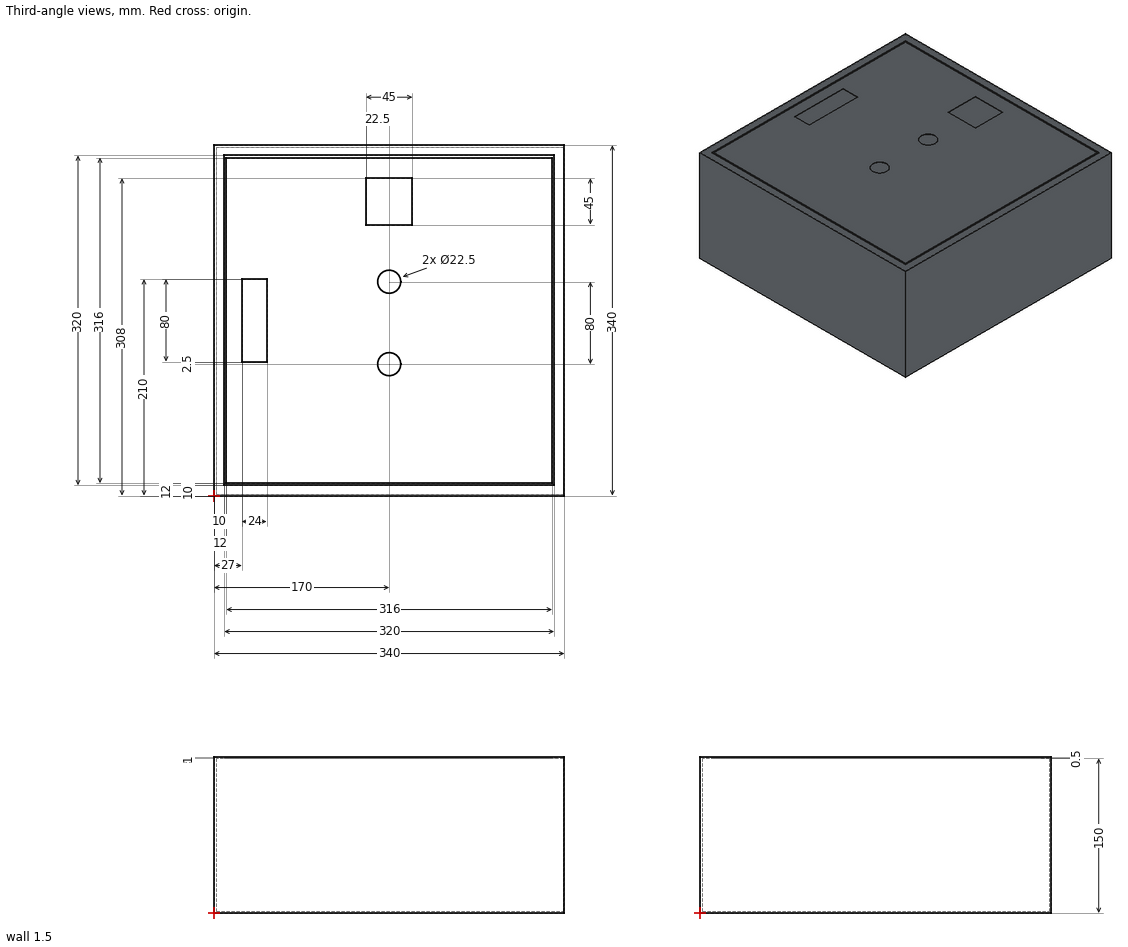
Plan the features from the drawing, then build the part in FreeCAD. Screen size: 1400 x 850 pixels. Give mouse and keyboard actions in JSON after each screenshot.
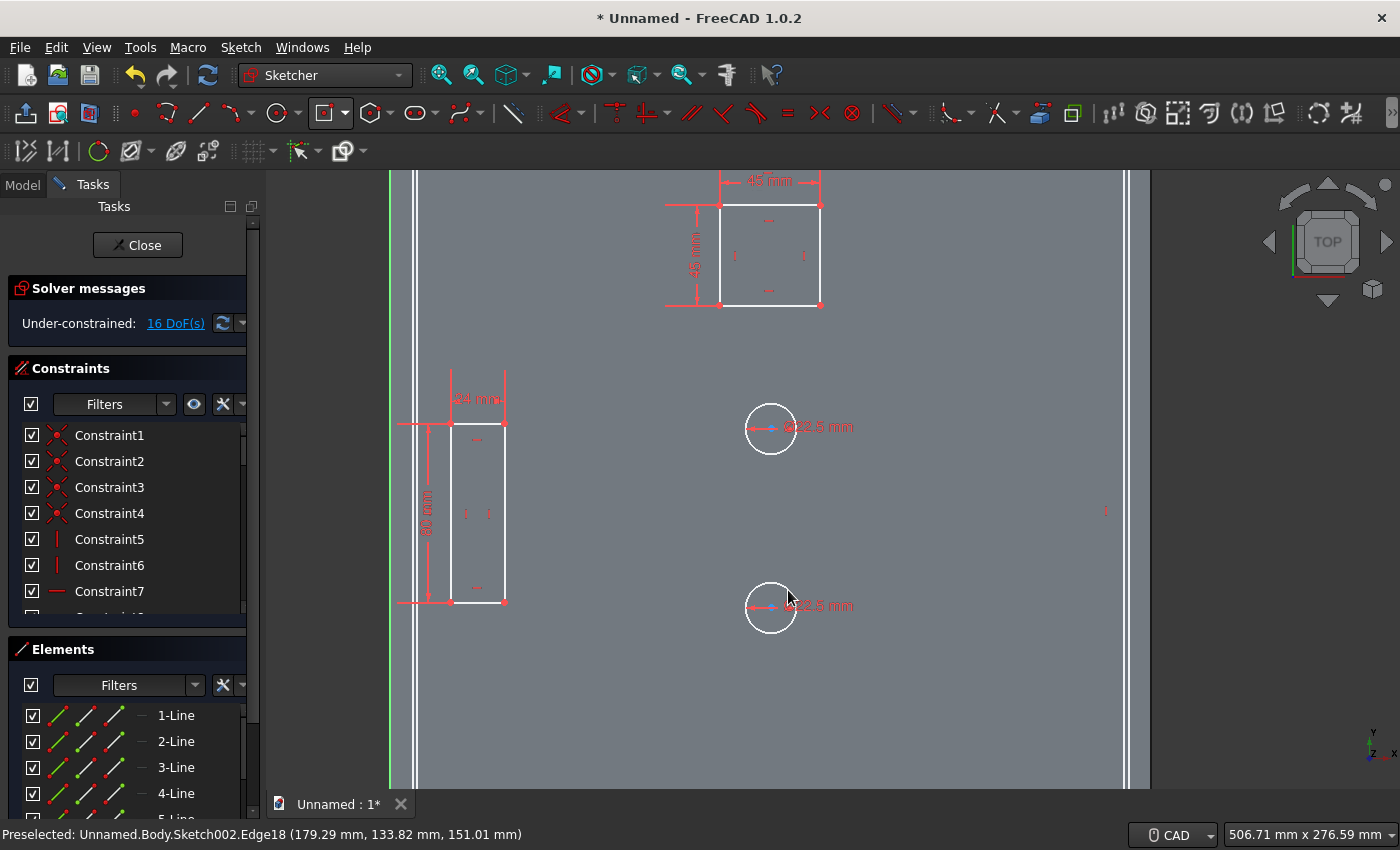
{"action": "left_click", "coordinate": [771, 429]}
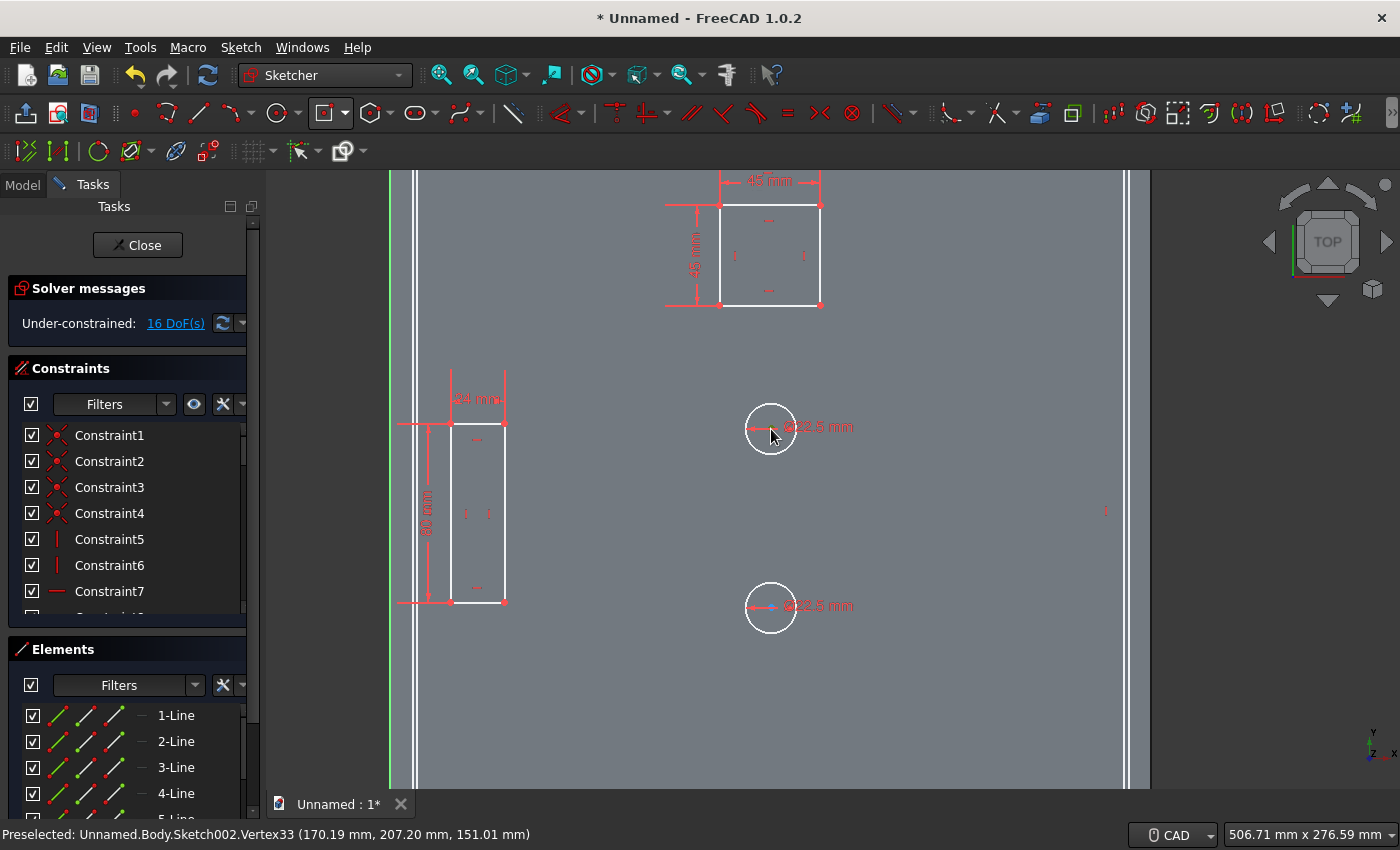
{"action": "left_click", "coordinate": [771, 608]}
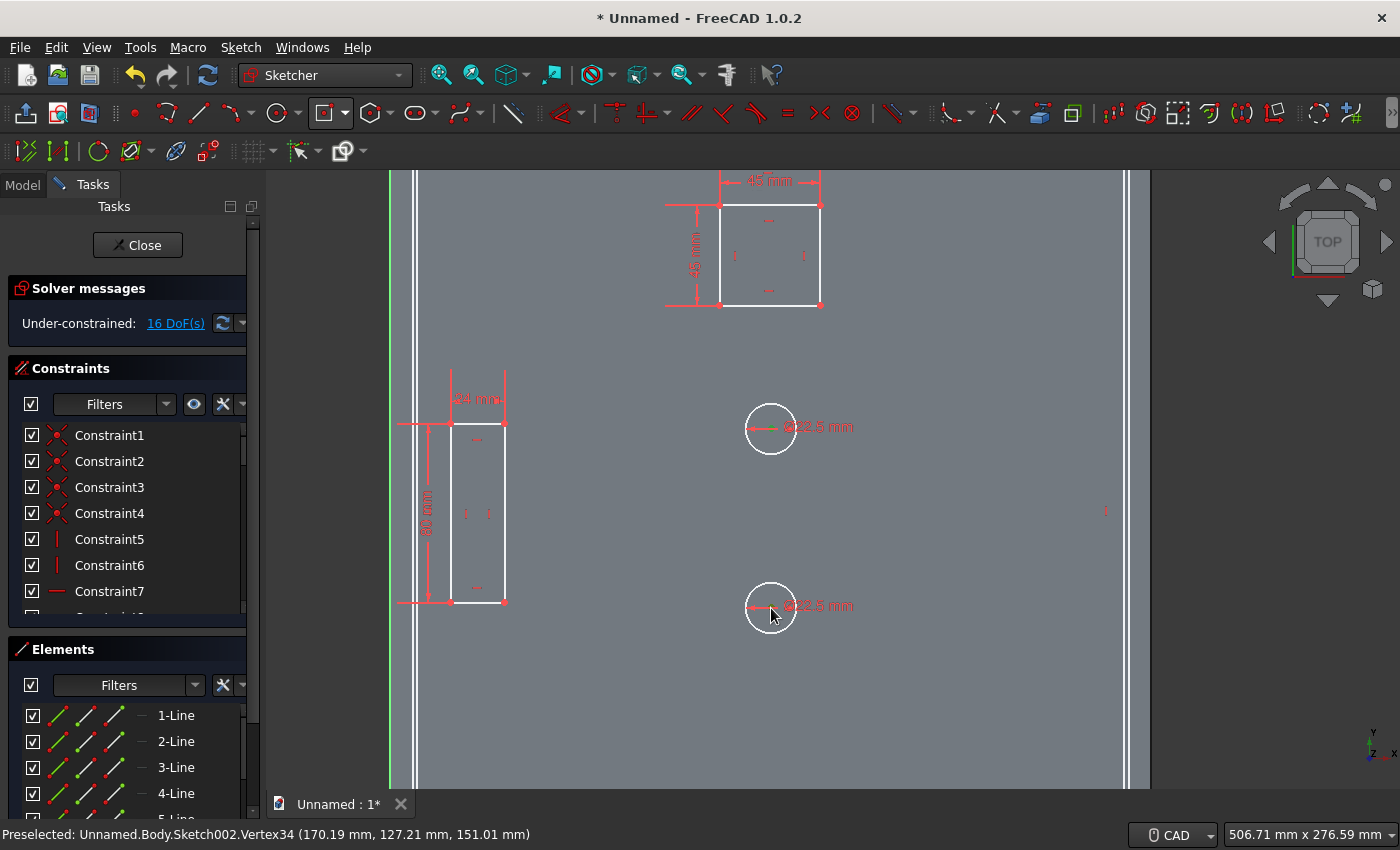
{"action": "key", "text": "v"}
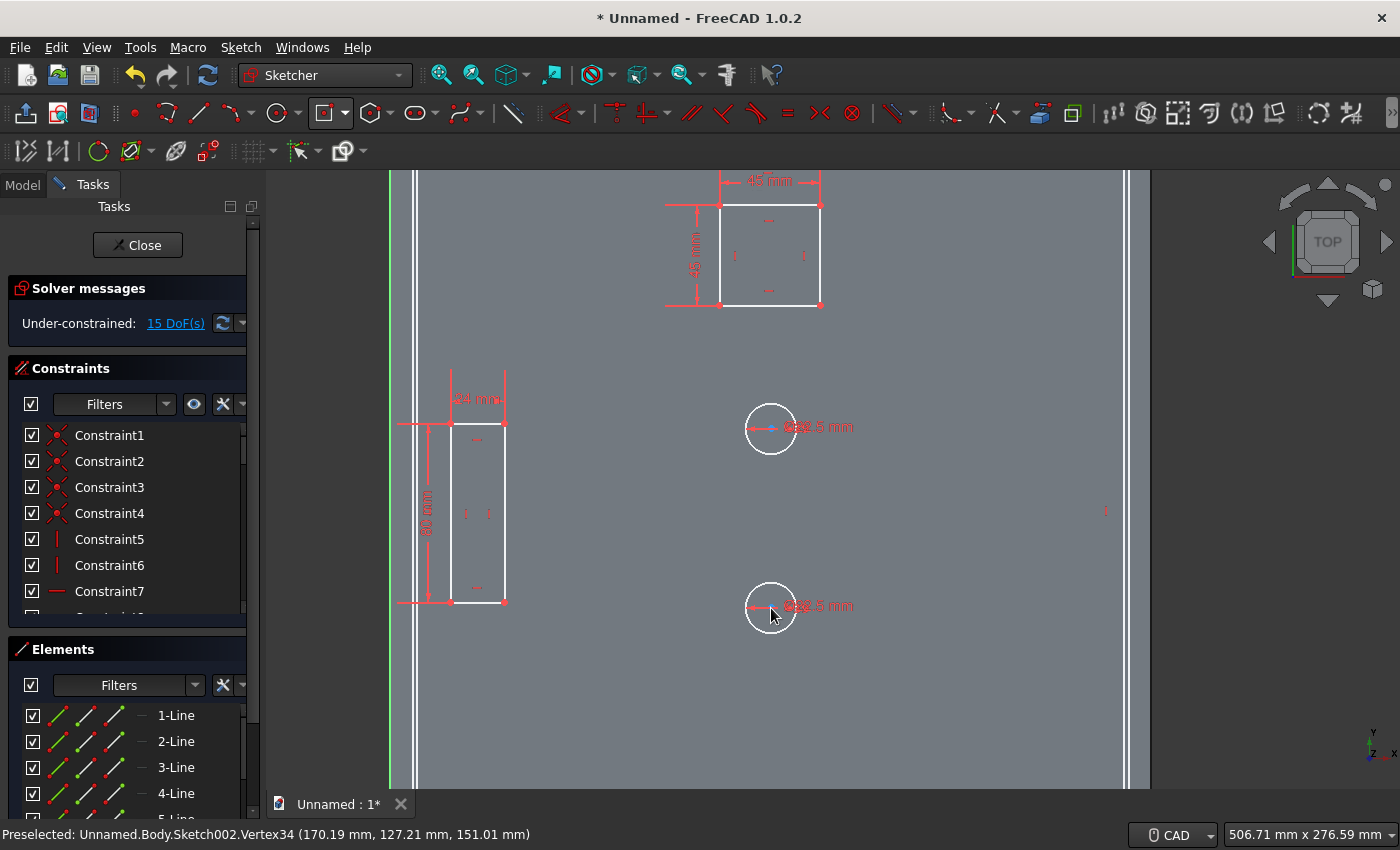
{"action": "scroll", "coordinate": [413, 370], "scroll_direction": "up", "scroll_amount": 7}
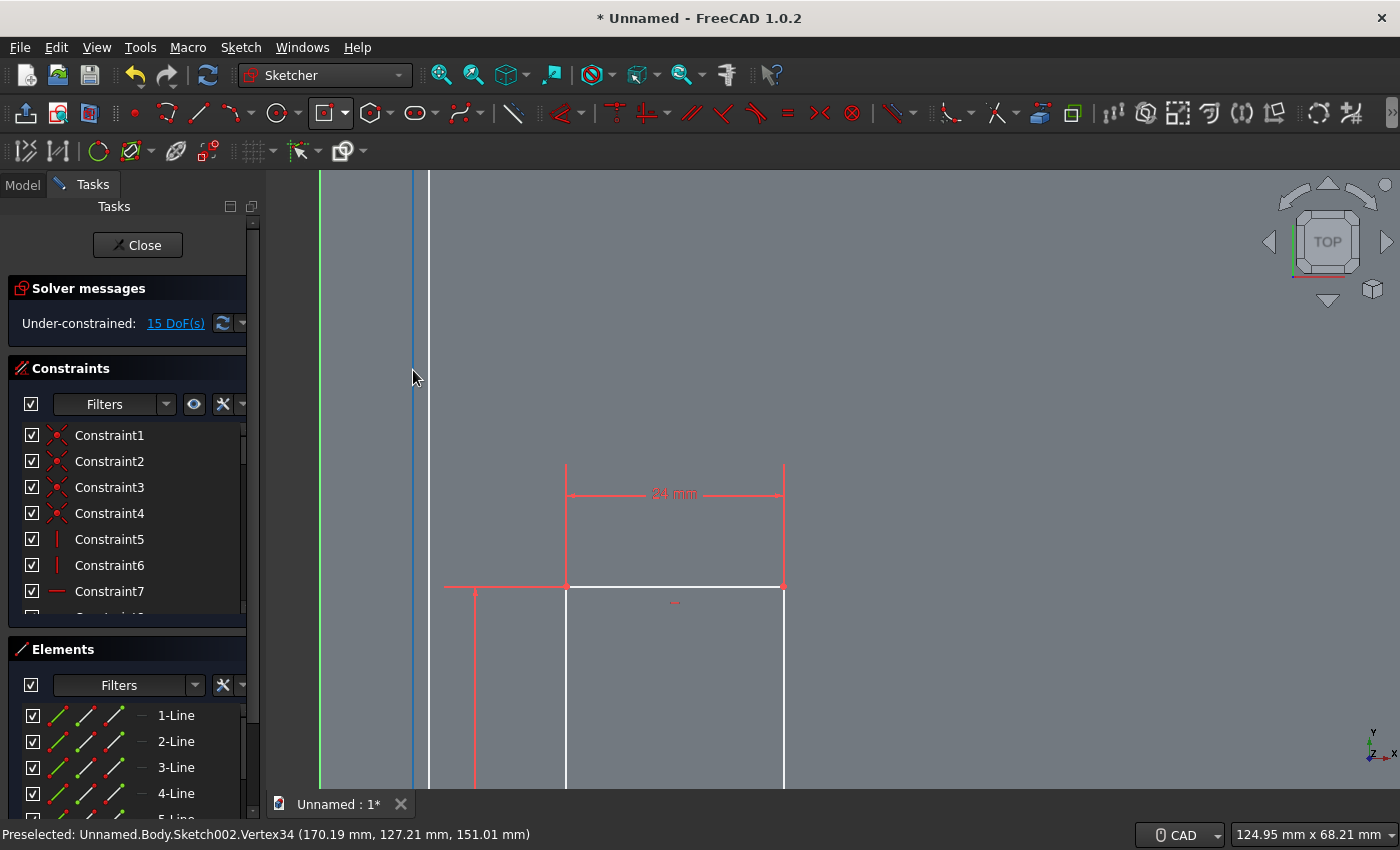
{"action": "left_click", "coordinate": [413, 371]}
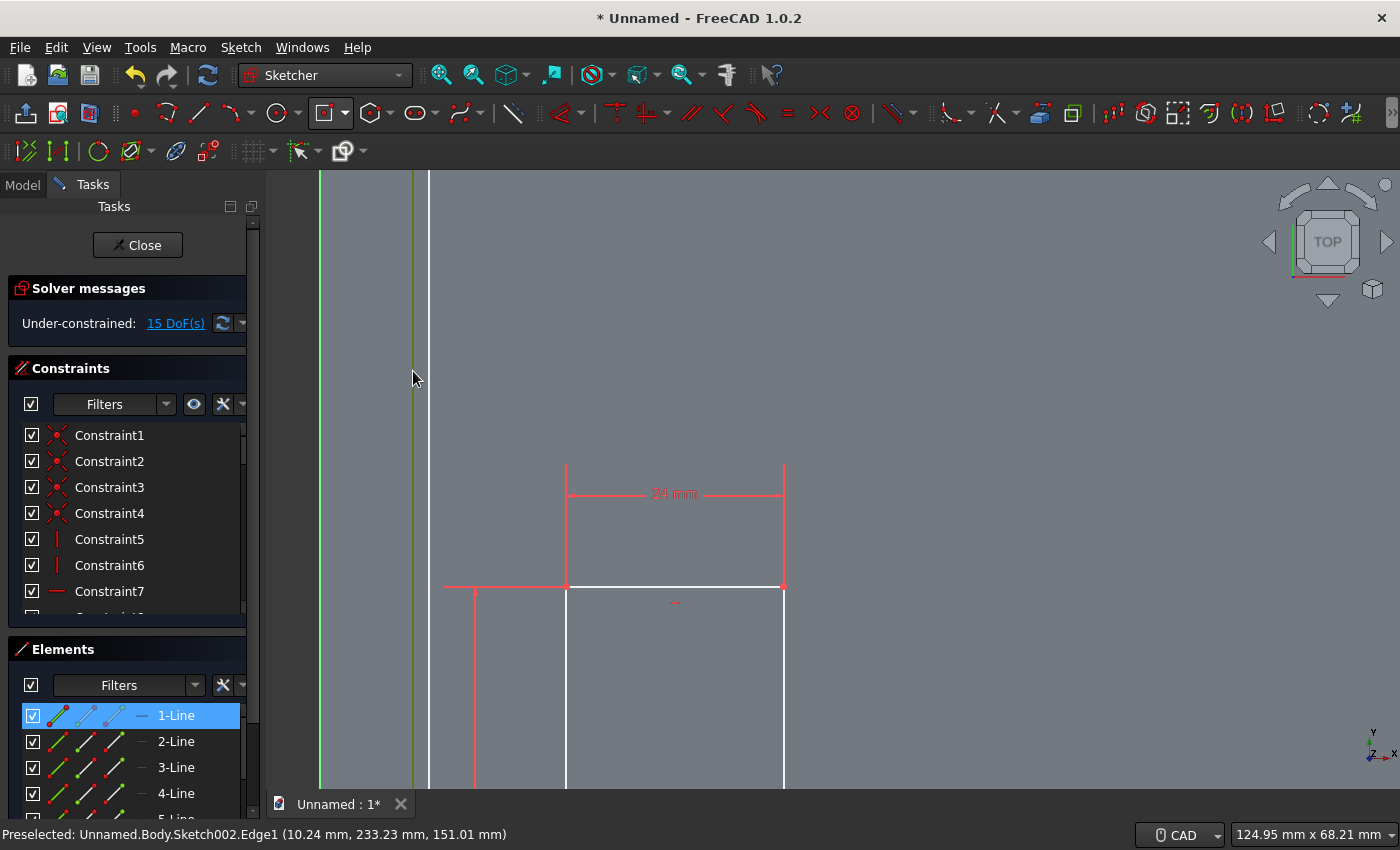
{"action": "key", "text": "i"}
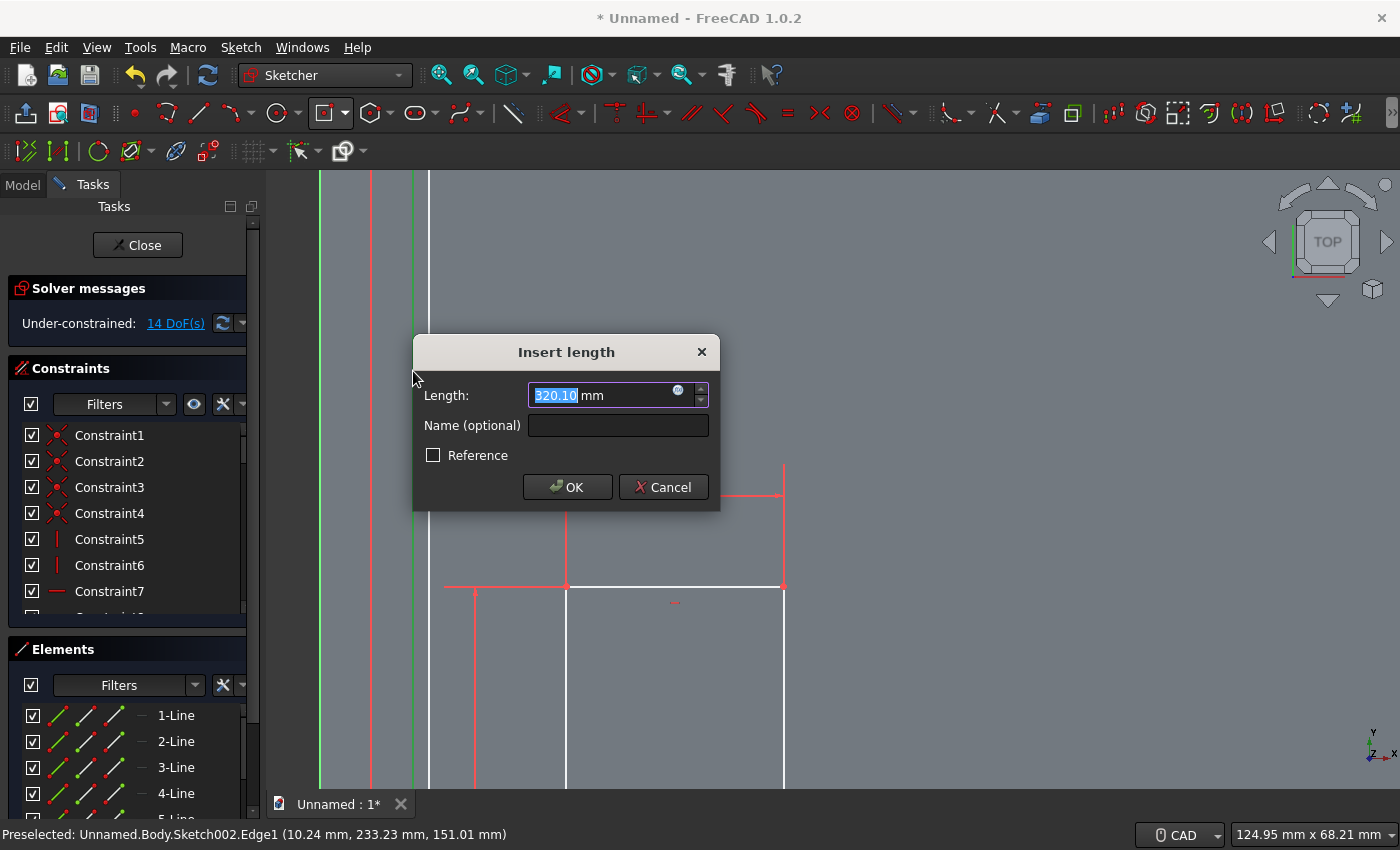
{"action": "type", "text": "320"}
{"action": "key", "text": "Return"}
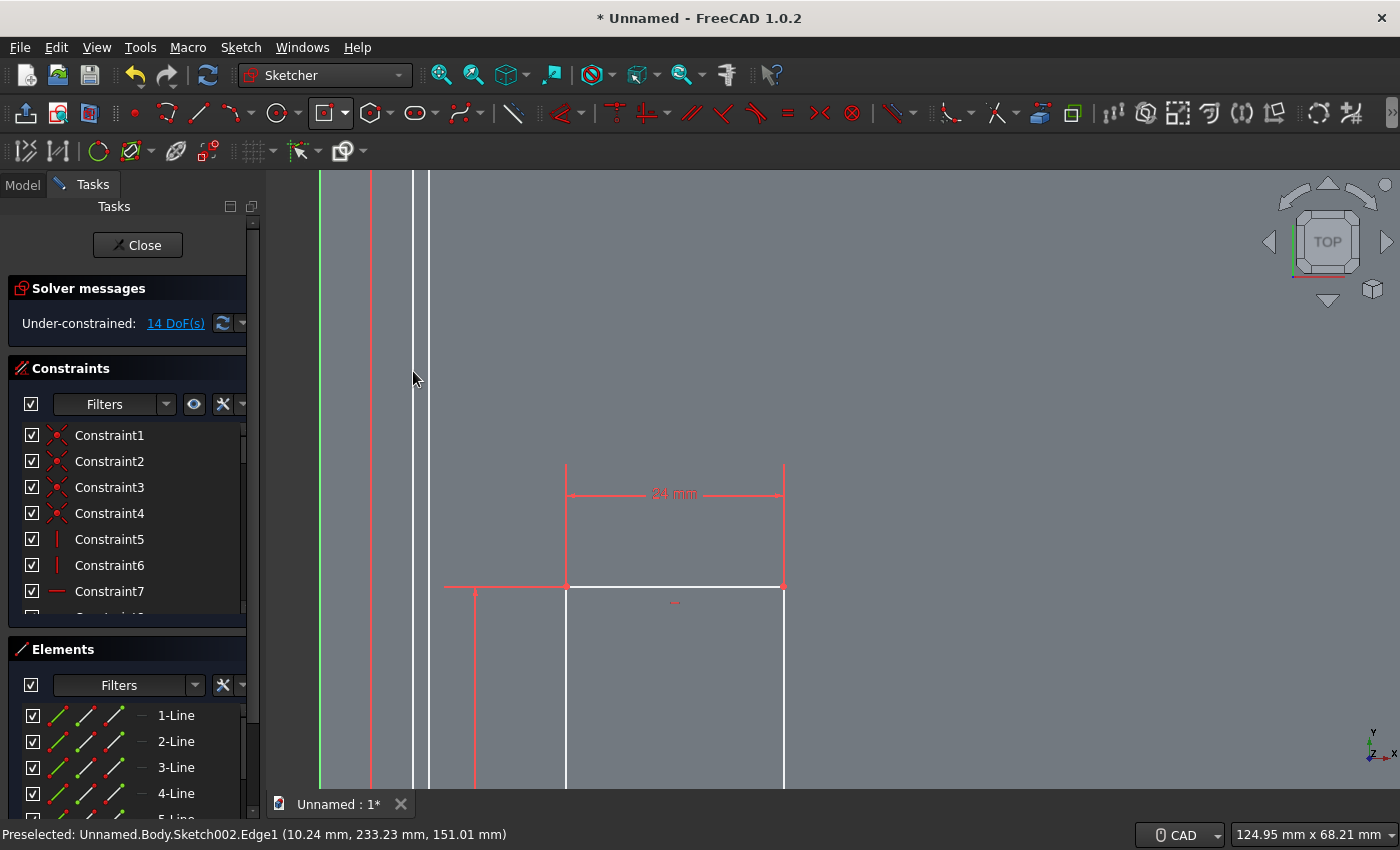
{"action": "scroll", "coordinate": [600, 399], "scroll_direction": "down", "scroll_amount": 10}